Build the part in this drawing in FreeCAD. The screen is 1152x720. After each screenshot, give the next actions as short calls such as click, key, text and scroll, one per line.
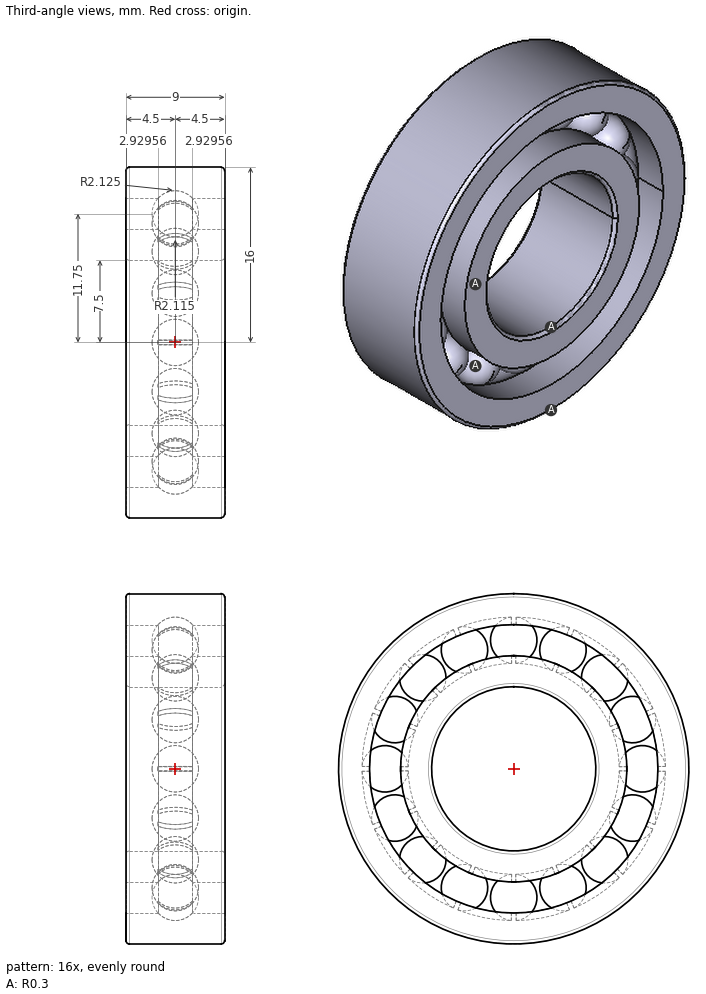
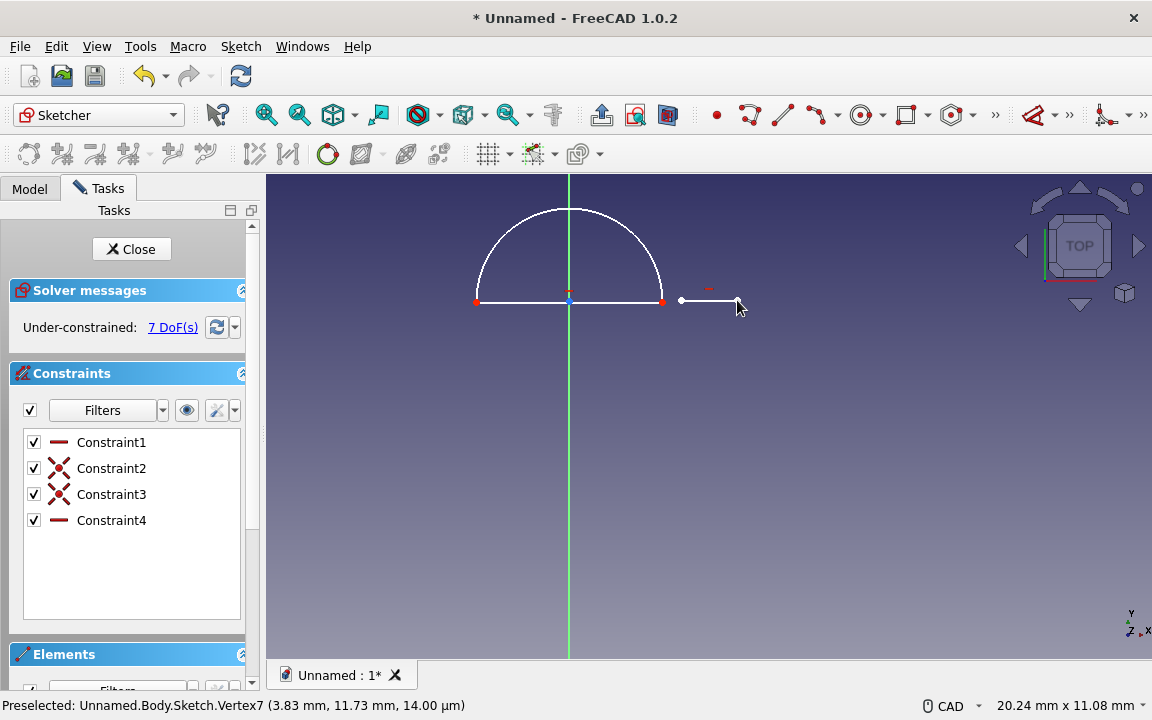
click(698, 301)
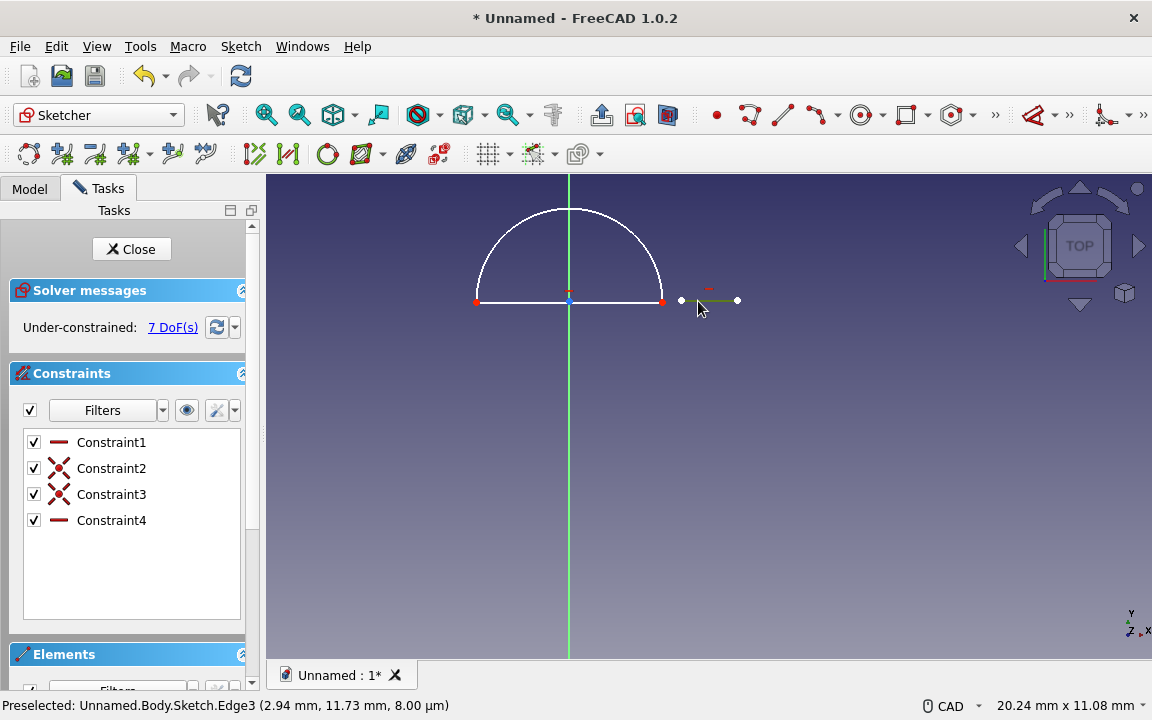
key(g)
key(n)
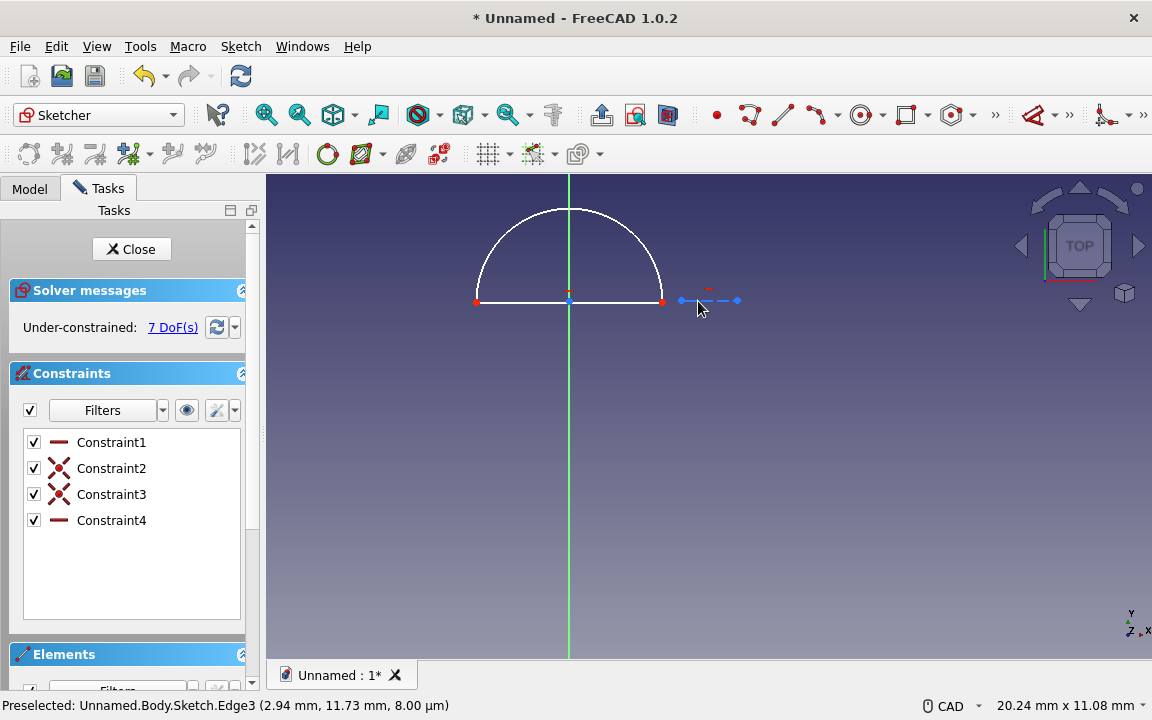
click(569, 302)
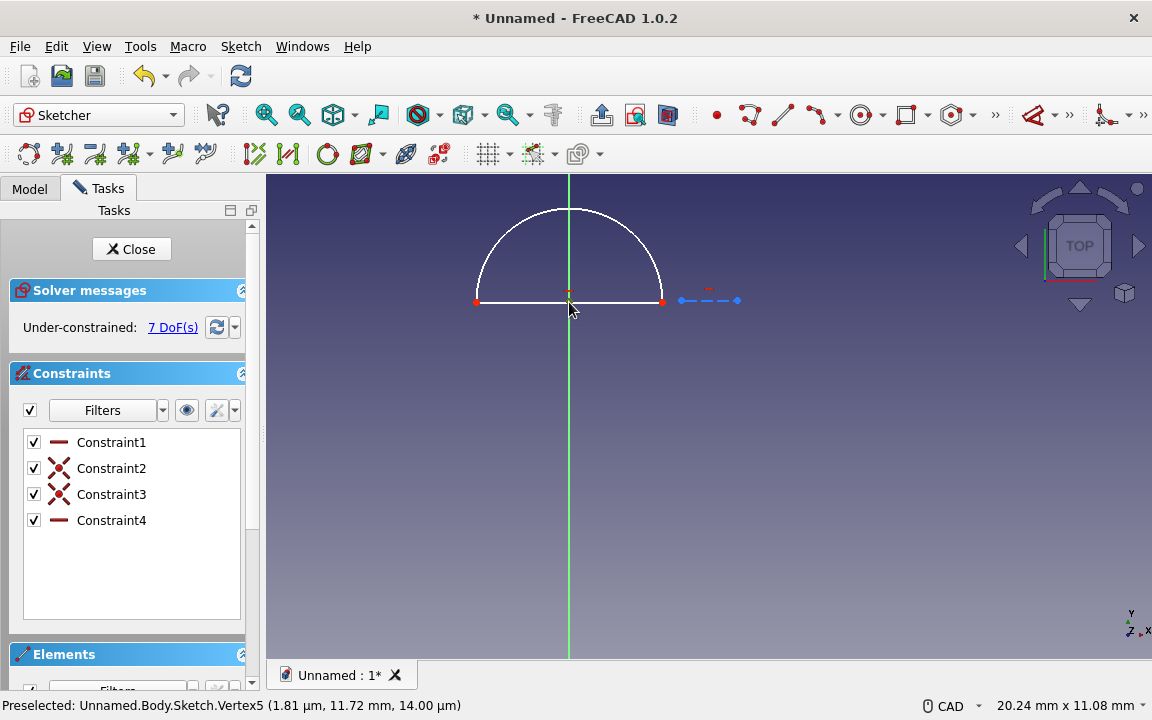
click(569, 600)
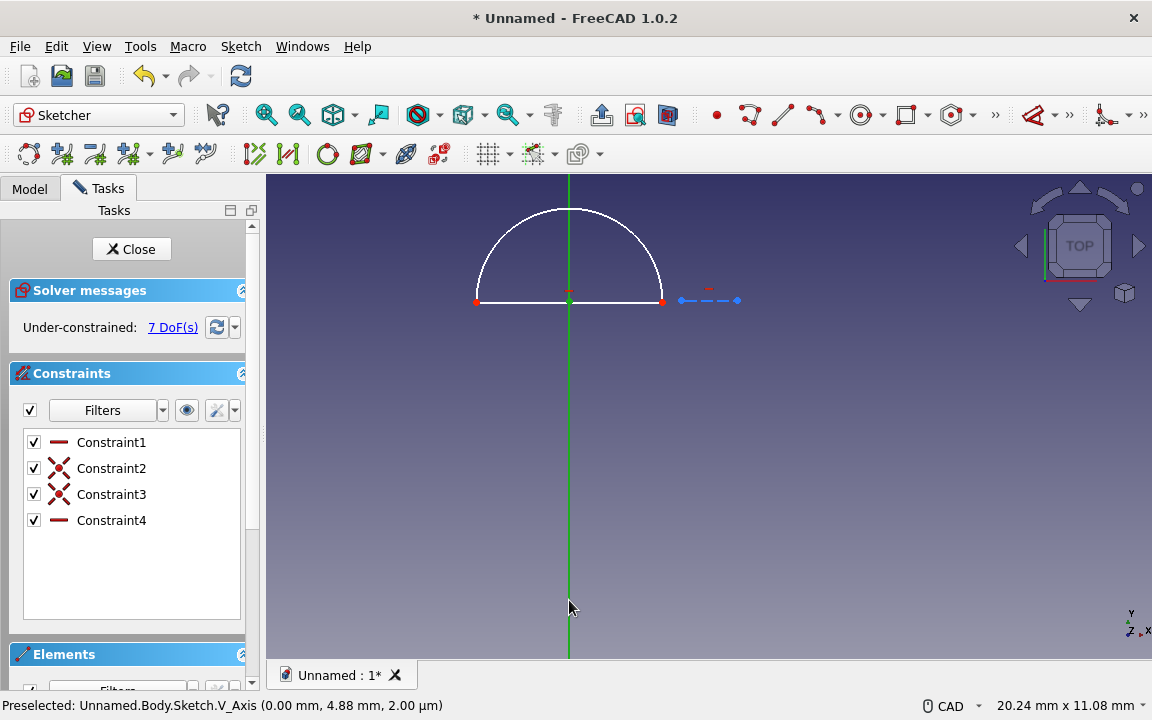
key(c)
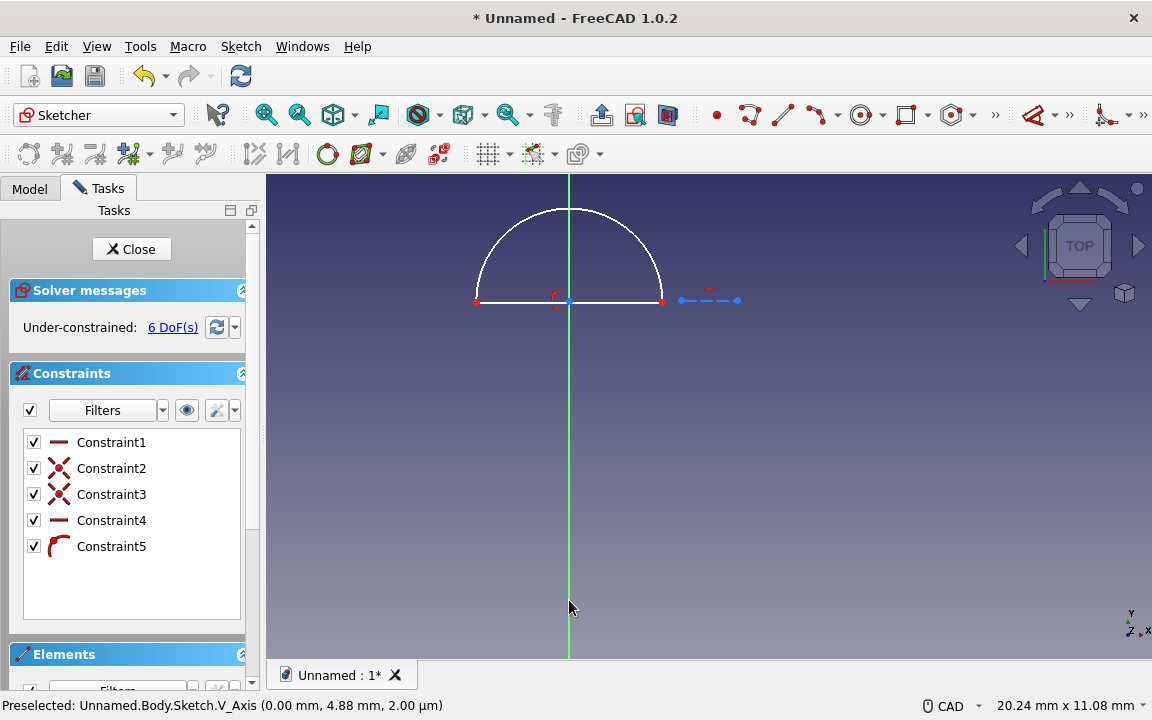
click(1032, 116)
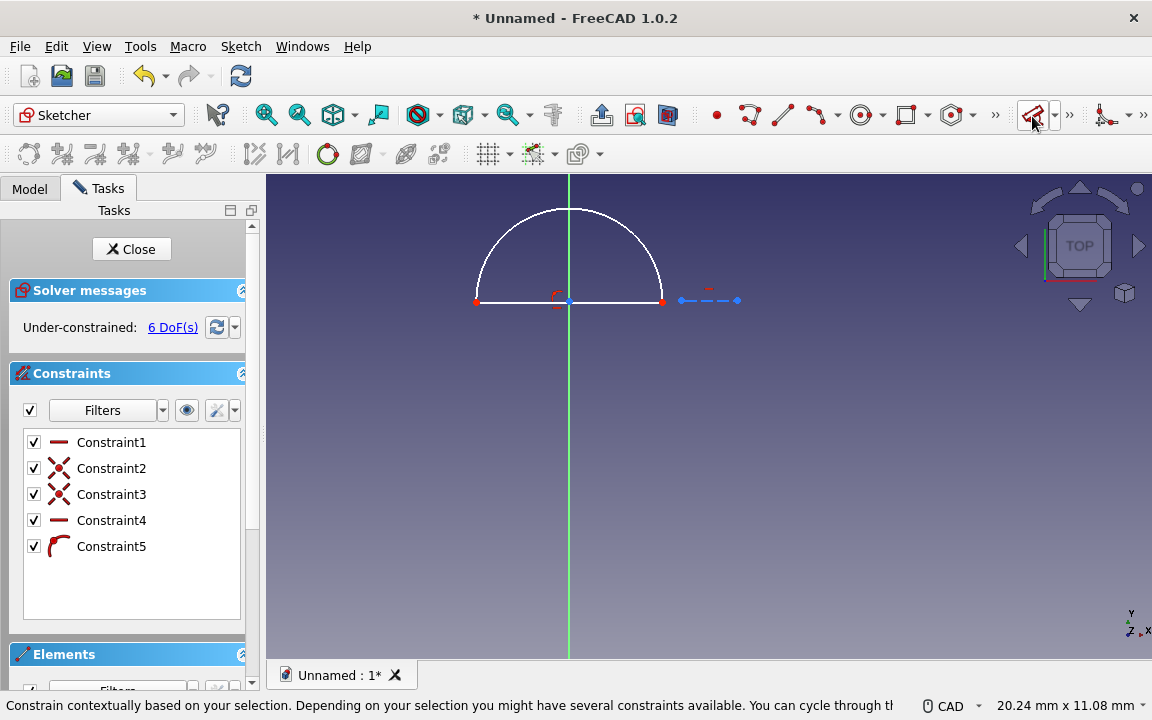
click(624, 227)
click(682, 249)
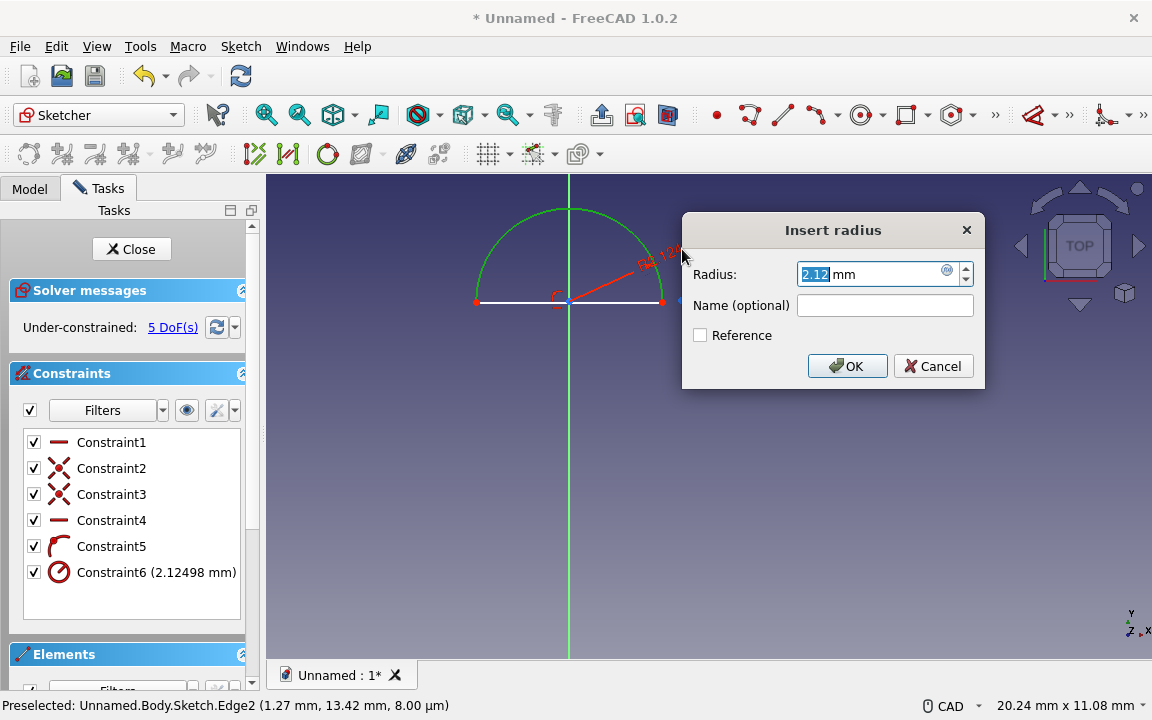
text(2.125)
key(Return)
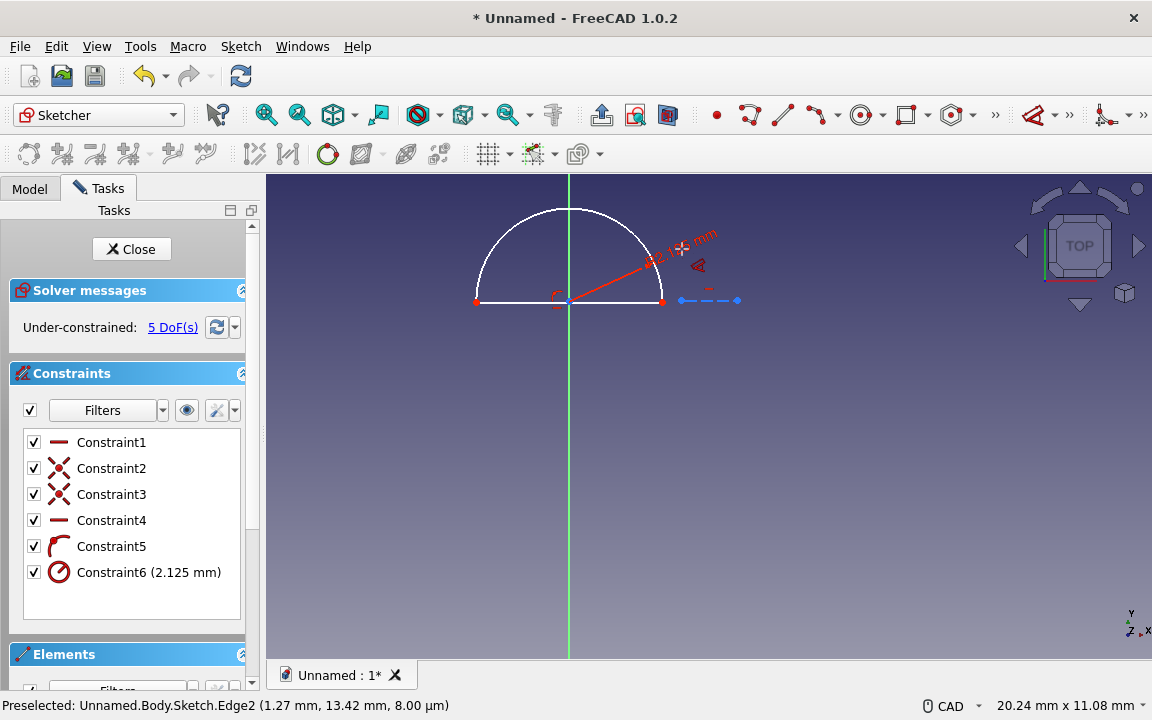
click(476, 303)
click(442, 467)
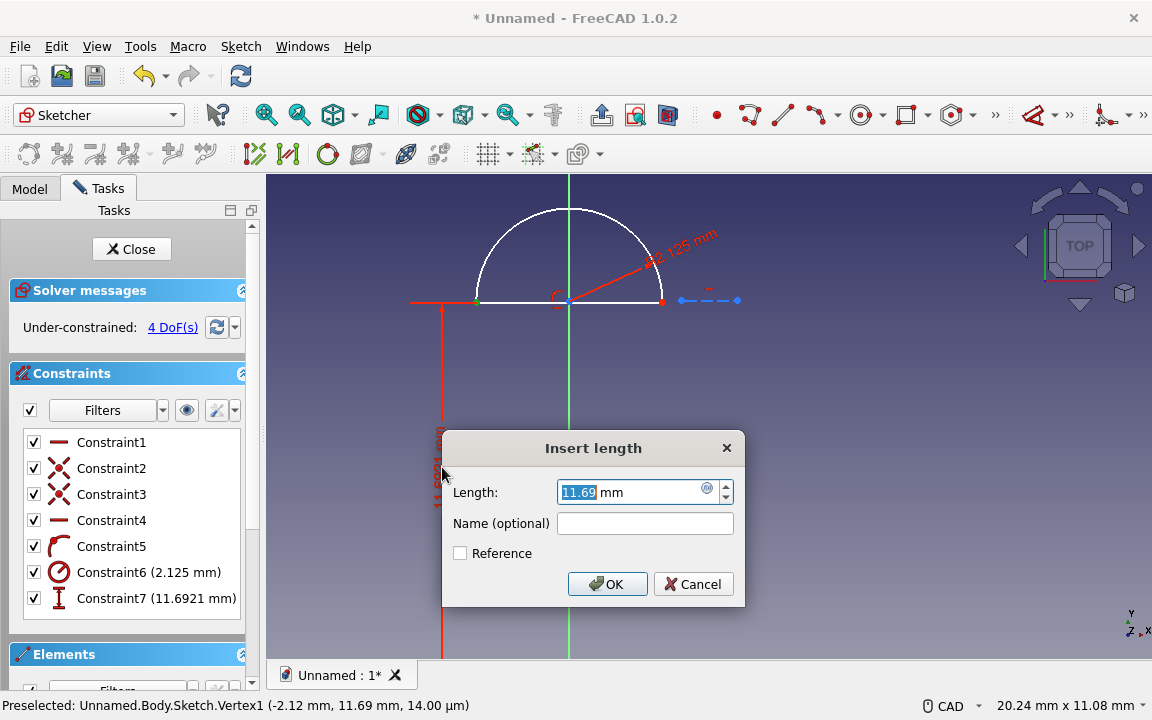
text(11.75)
key(Return)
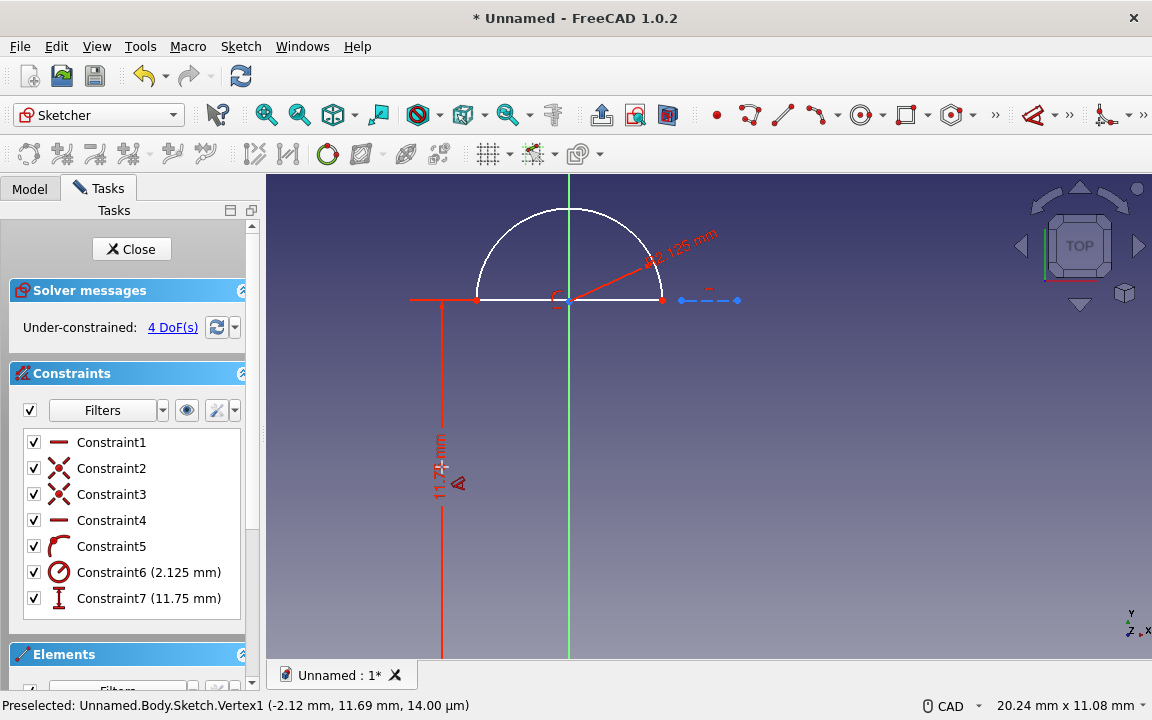
click(681, 301)
click(715, 466)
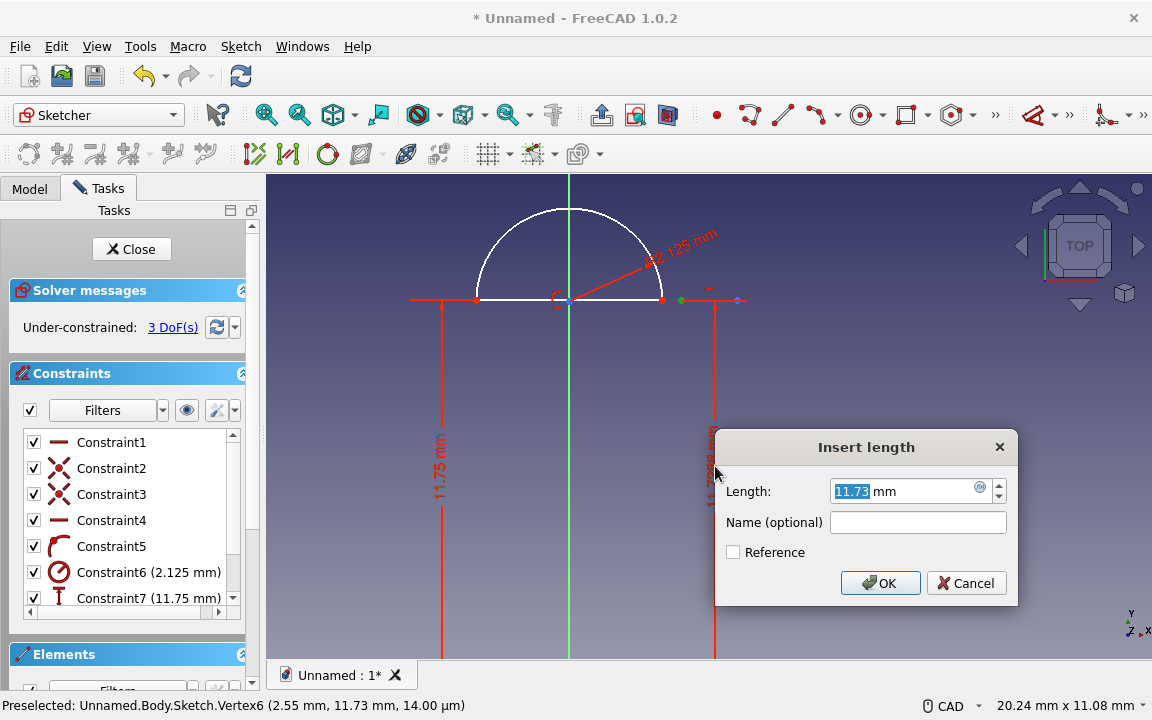
text(11.75)
key(Return)